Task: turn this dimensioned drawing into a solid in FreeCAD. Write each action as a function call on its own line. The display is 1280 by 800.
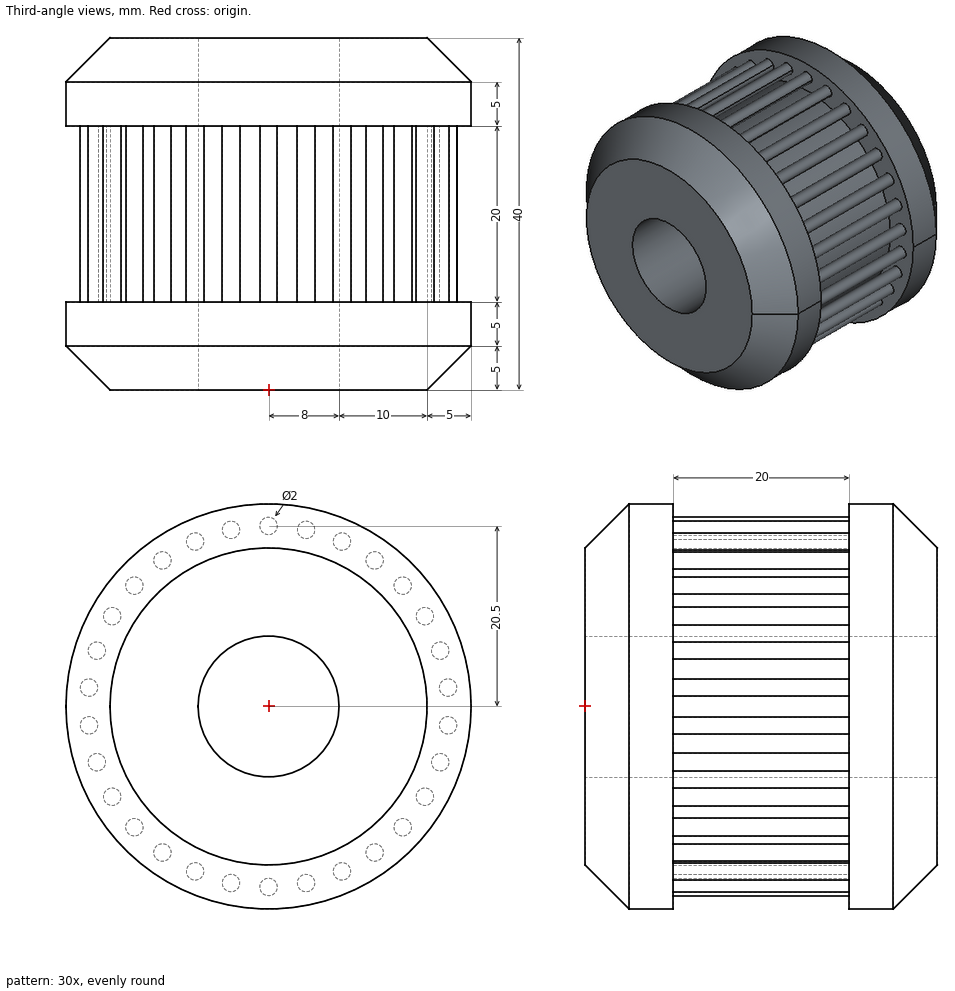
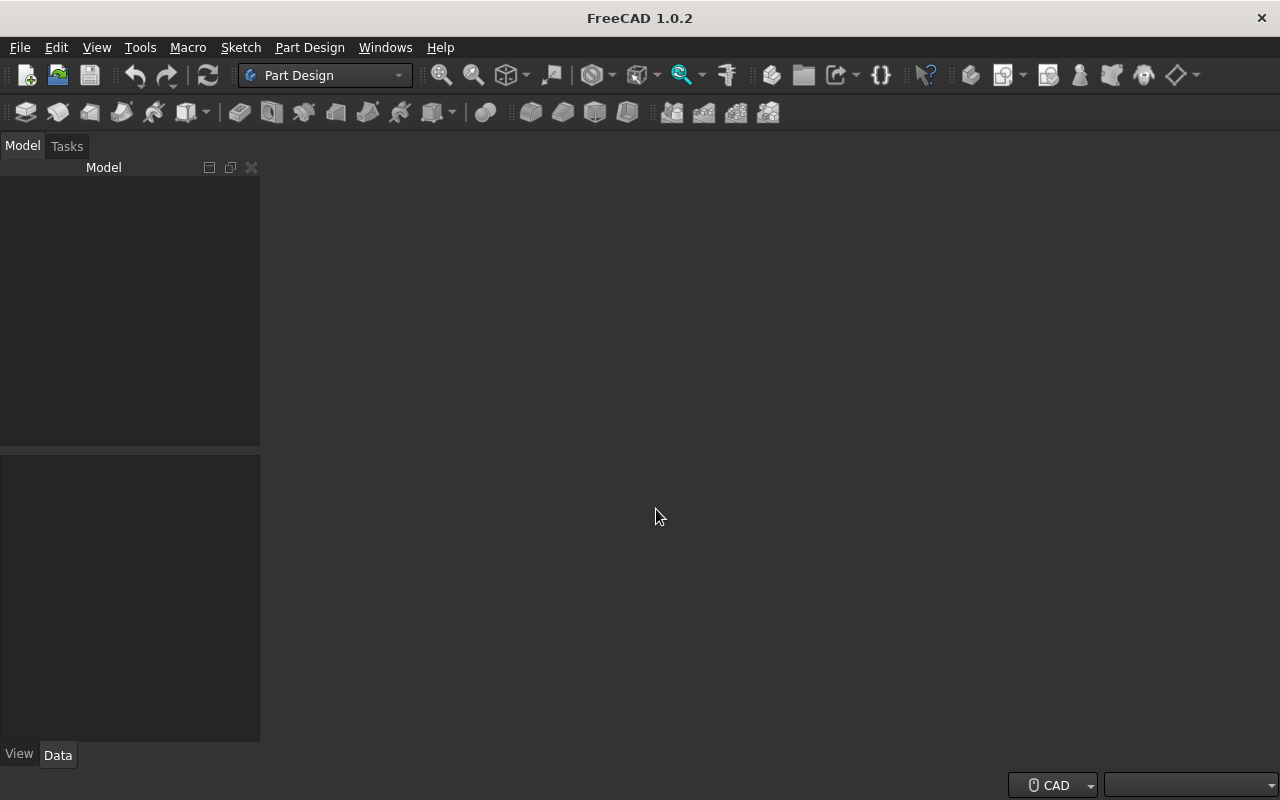
key(ctrl+n)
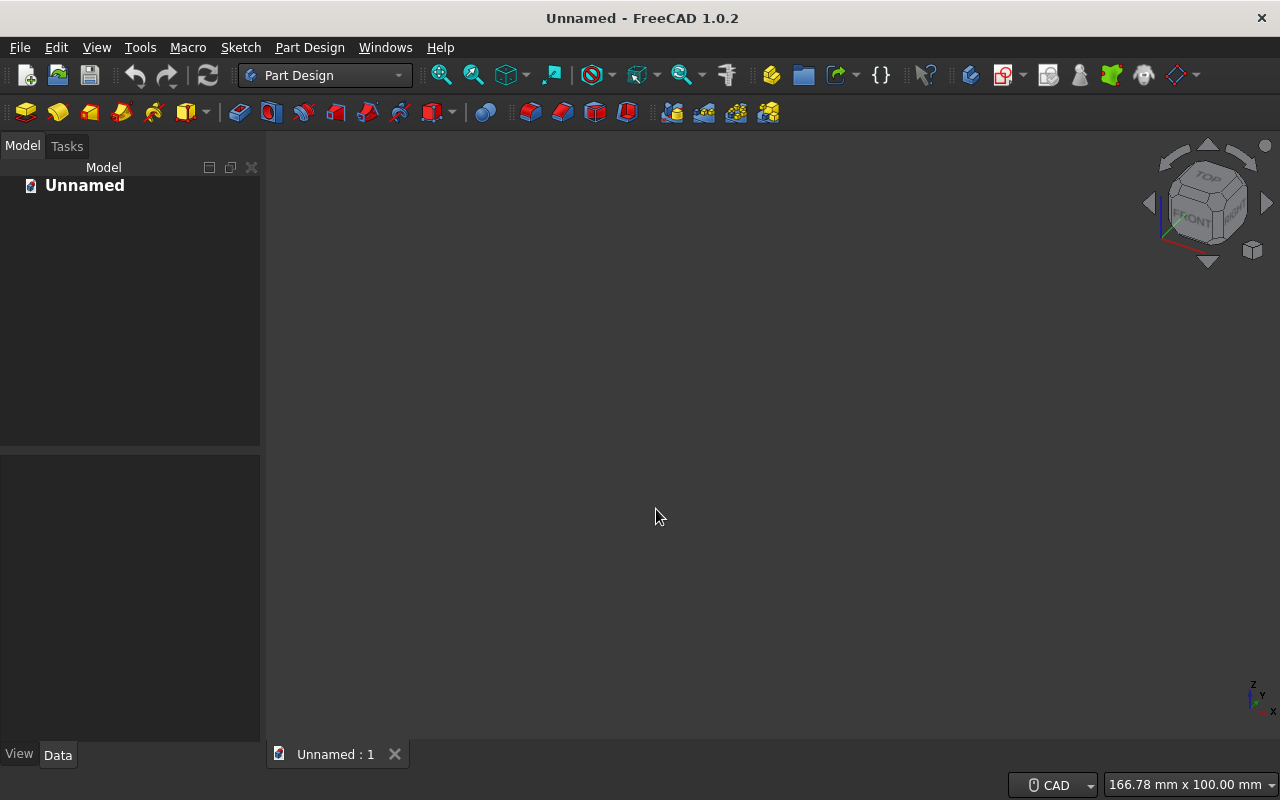
click(1004, 76)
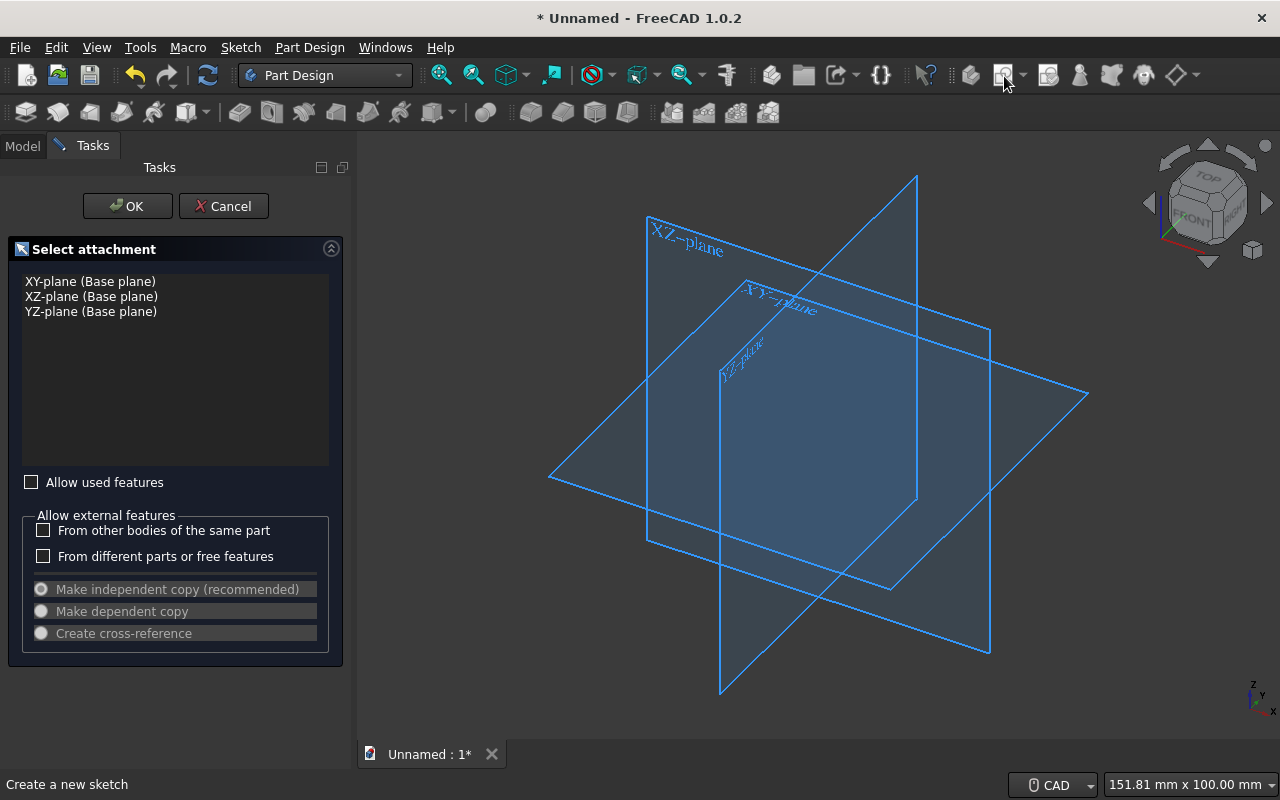
click(82, 282)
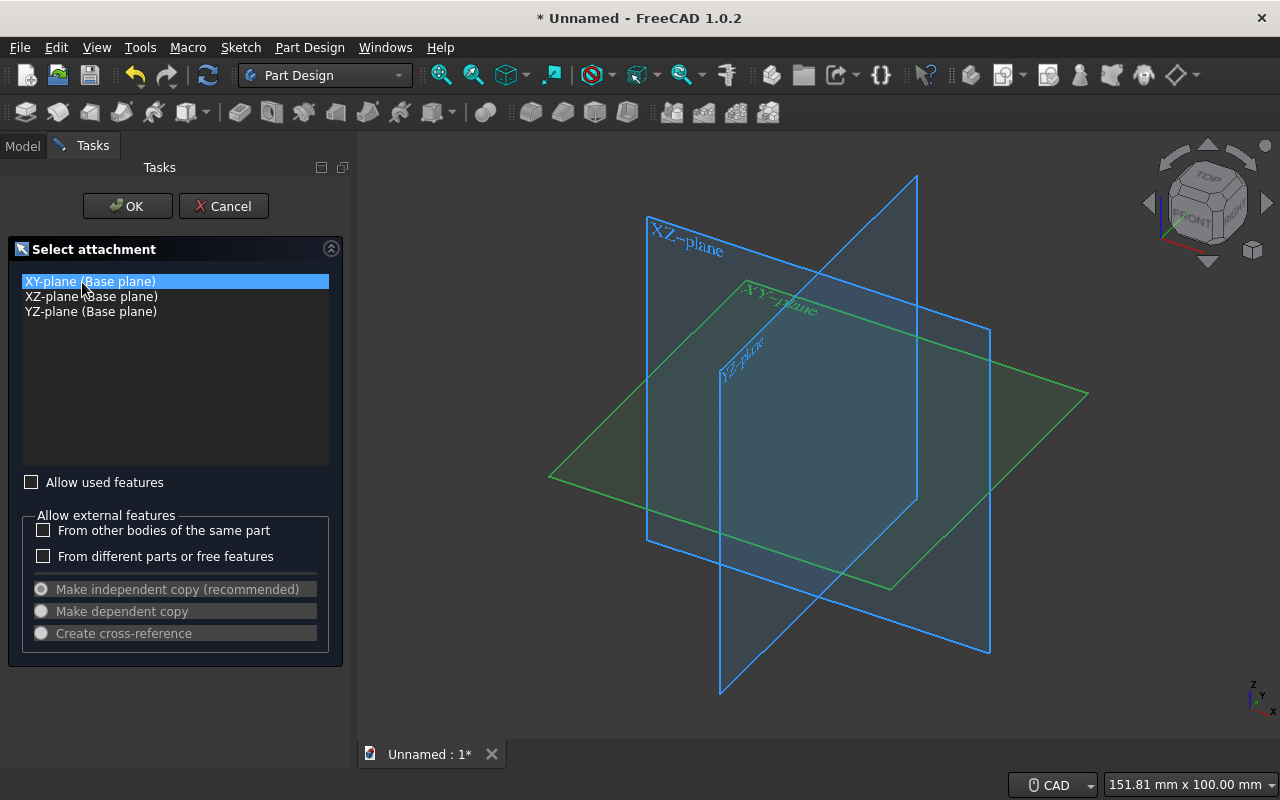
click(128, 206)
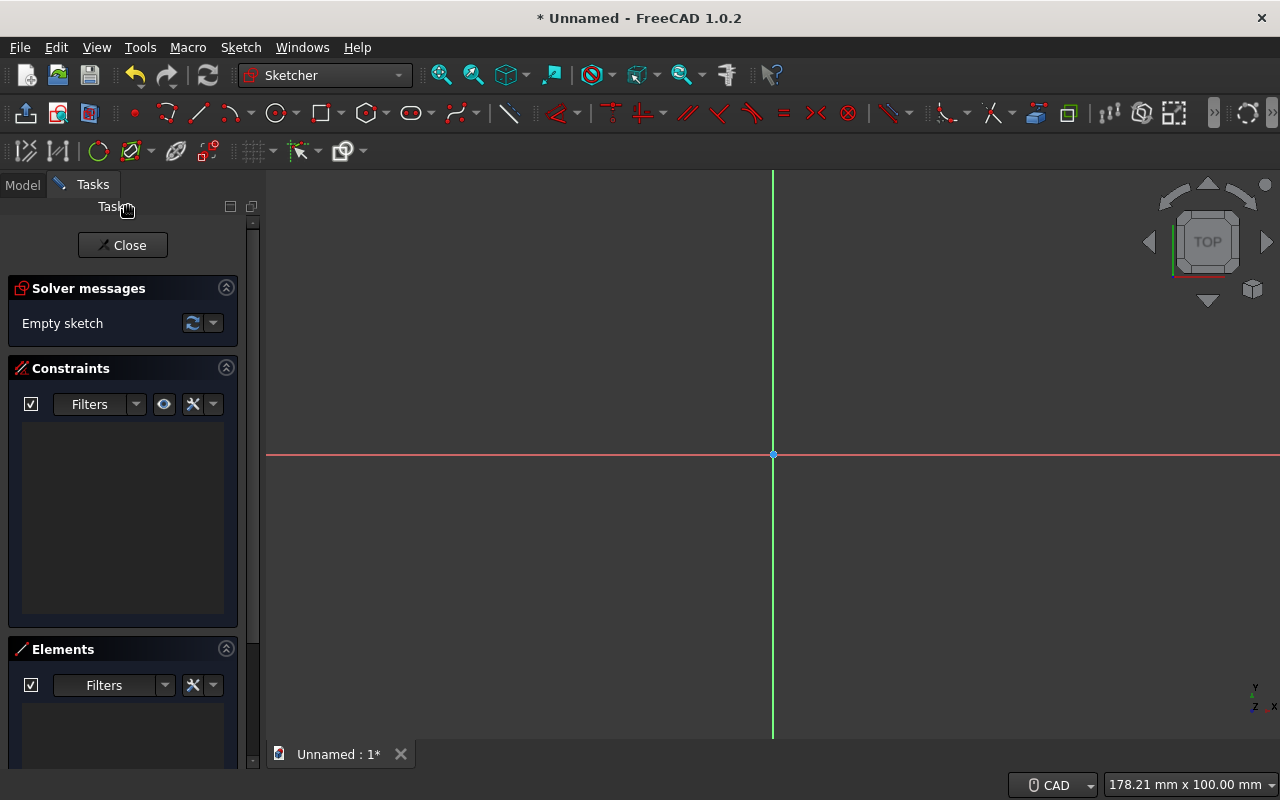
scroll(1111, 198, up, 2)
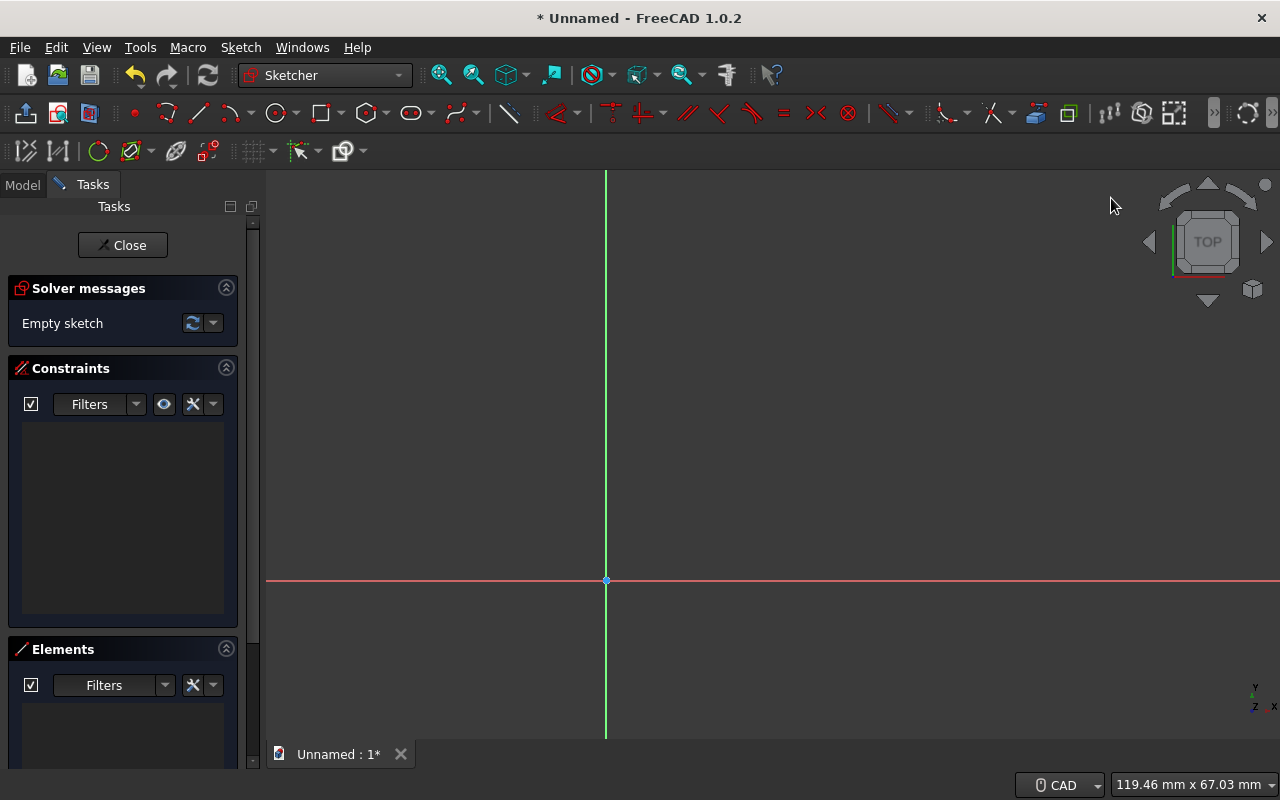
key(g)
key(m)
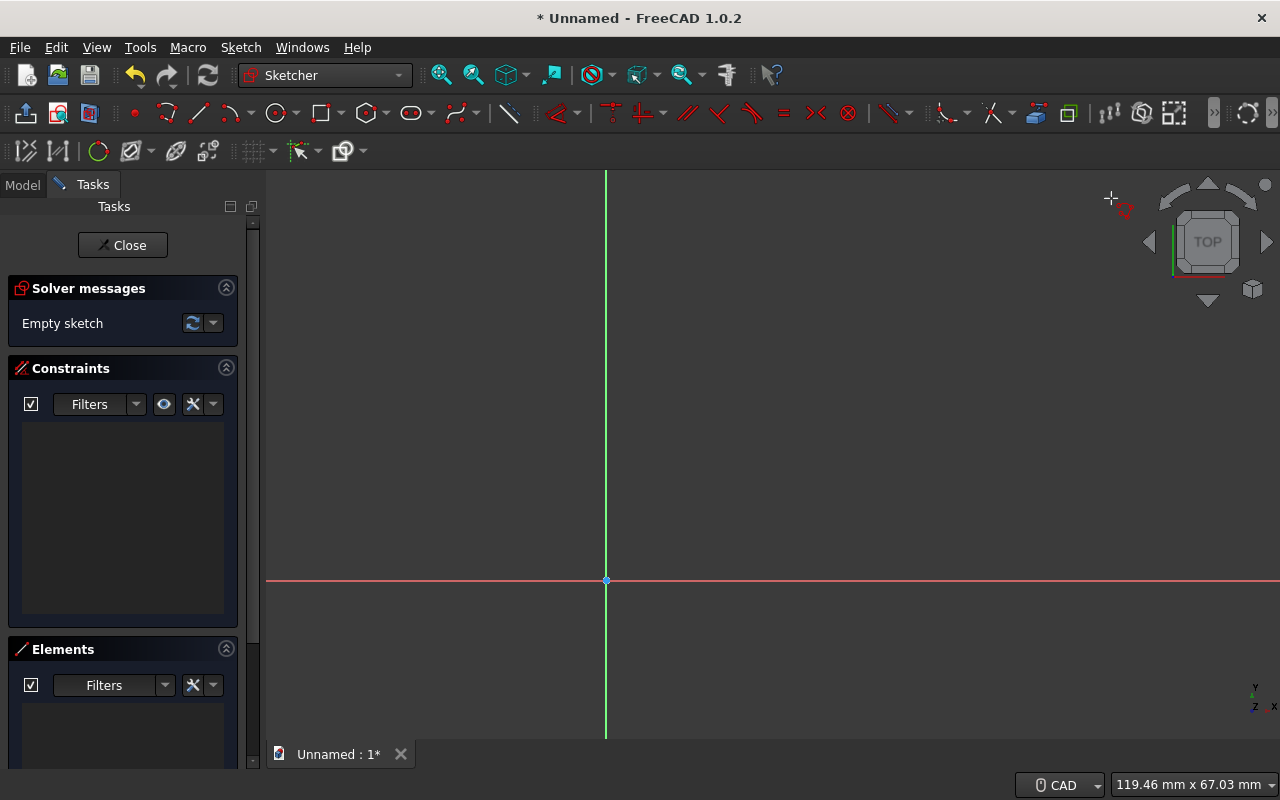
click(674, 581)
click(759, 572)
click(802, 538)
click(802, 496)
click(759, 496)
click(759, 326)
click(802, 326)
click(802, 284)
click(759, 241)
click(674, 241)
click(674, 581)
key(Escape)
key(Escape)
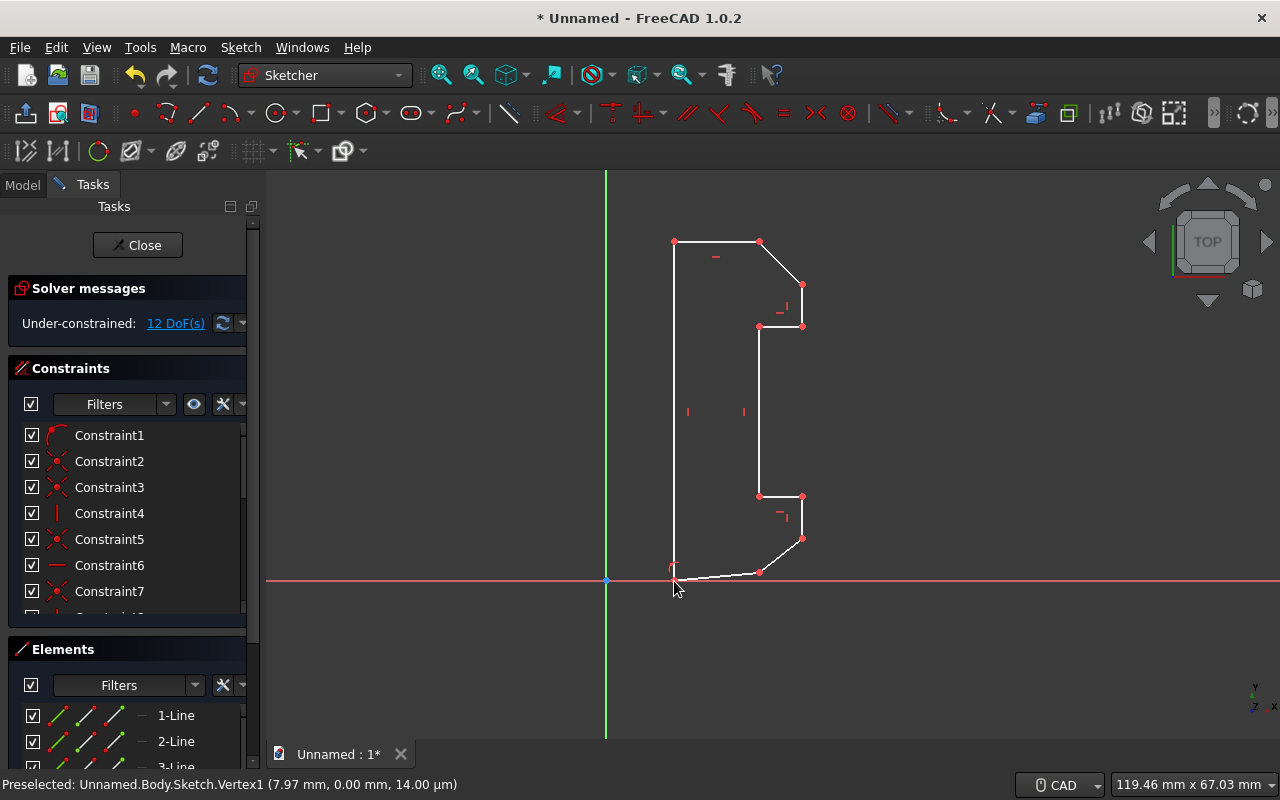
click(700, 578)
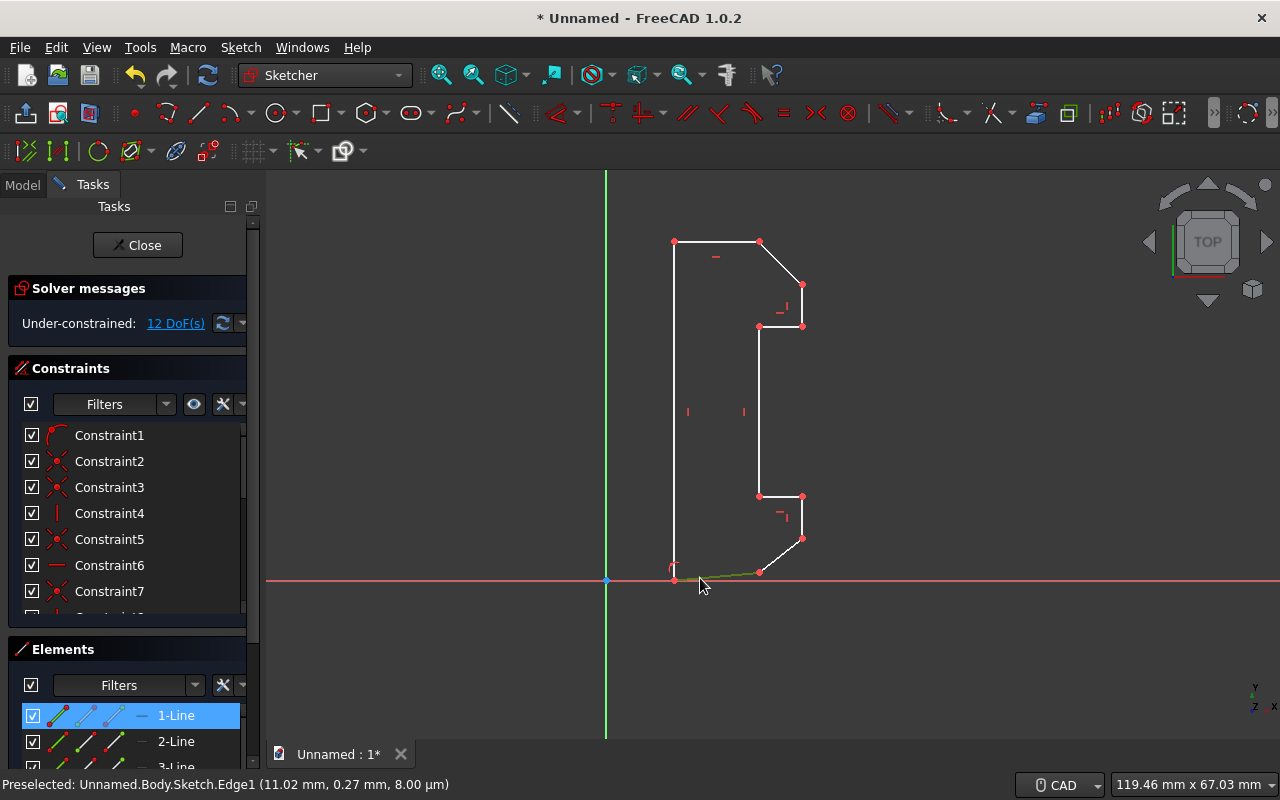
key(h)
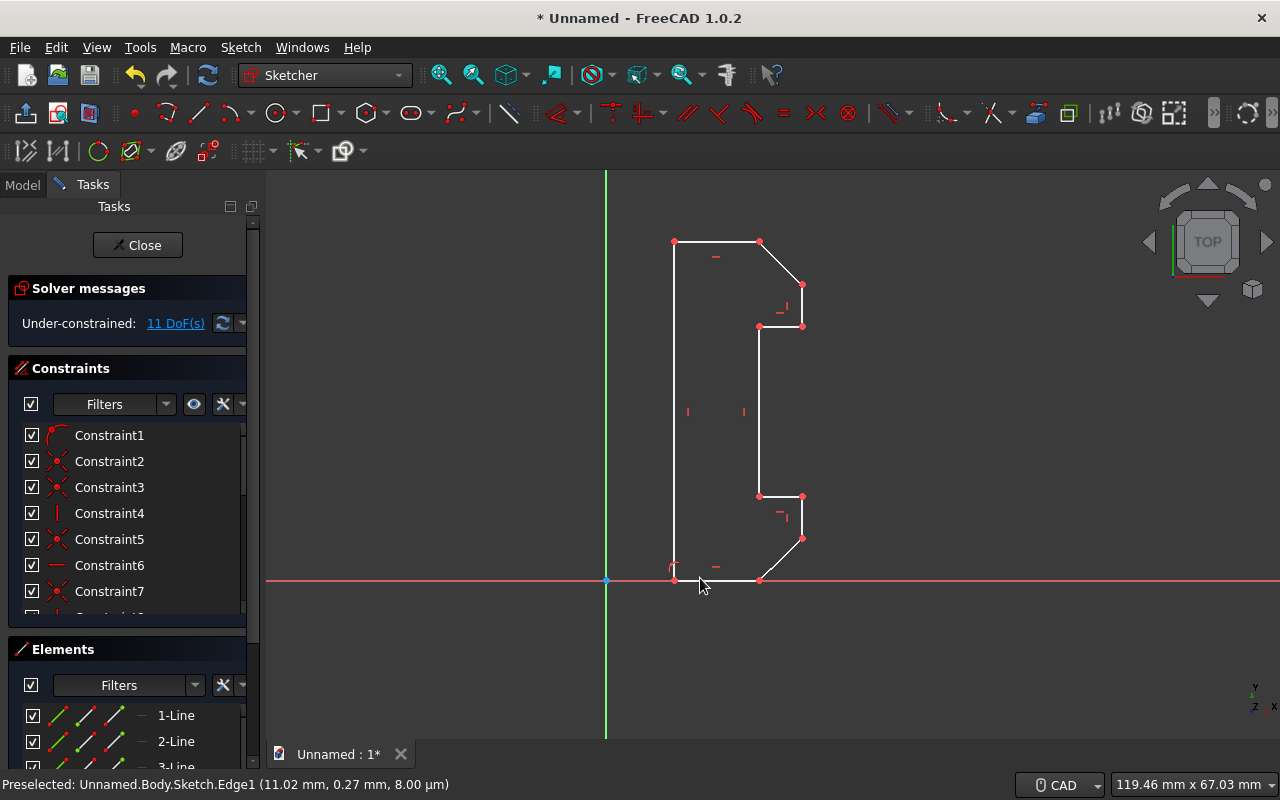
click(802, 526)